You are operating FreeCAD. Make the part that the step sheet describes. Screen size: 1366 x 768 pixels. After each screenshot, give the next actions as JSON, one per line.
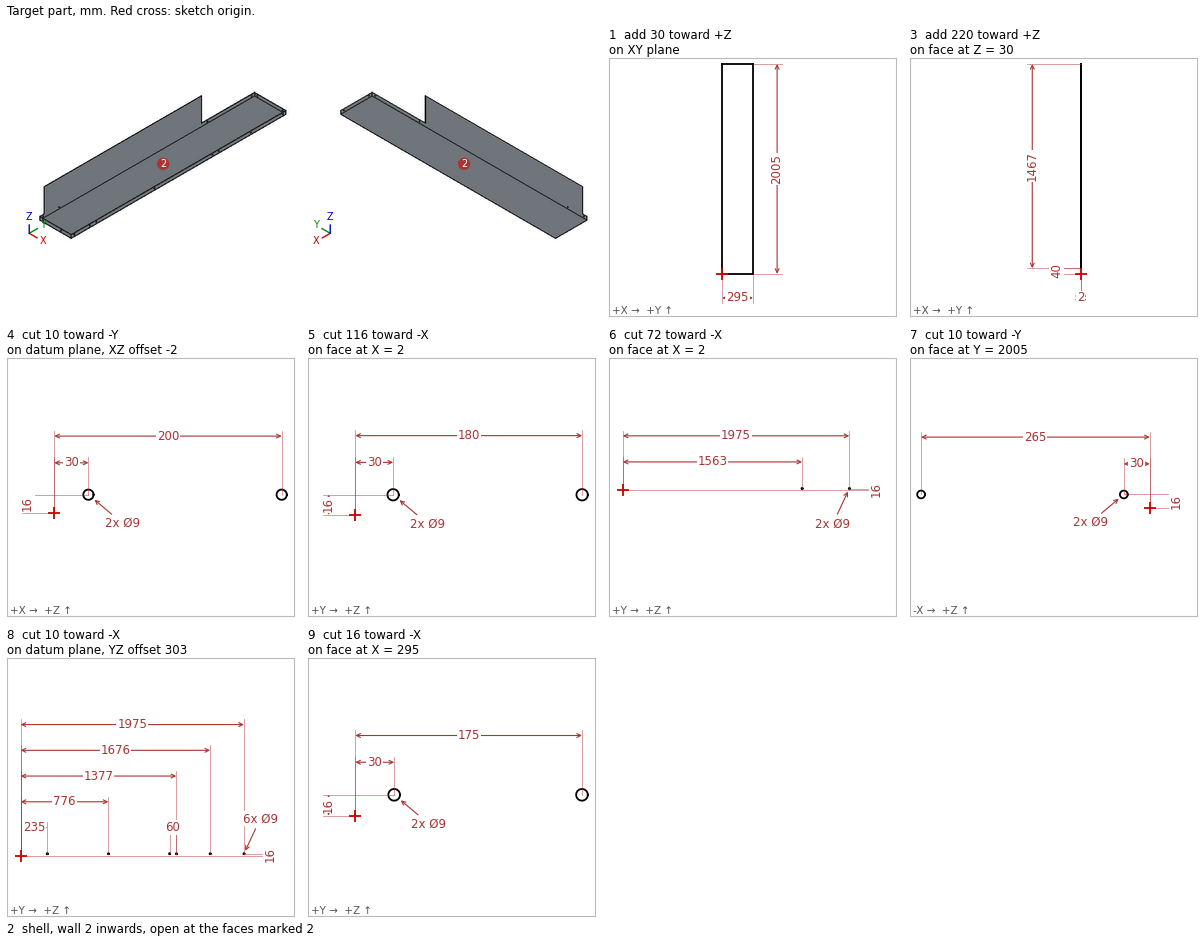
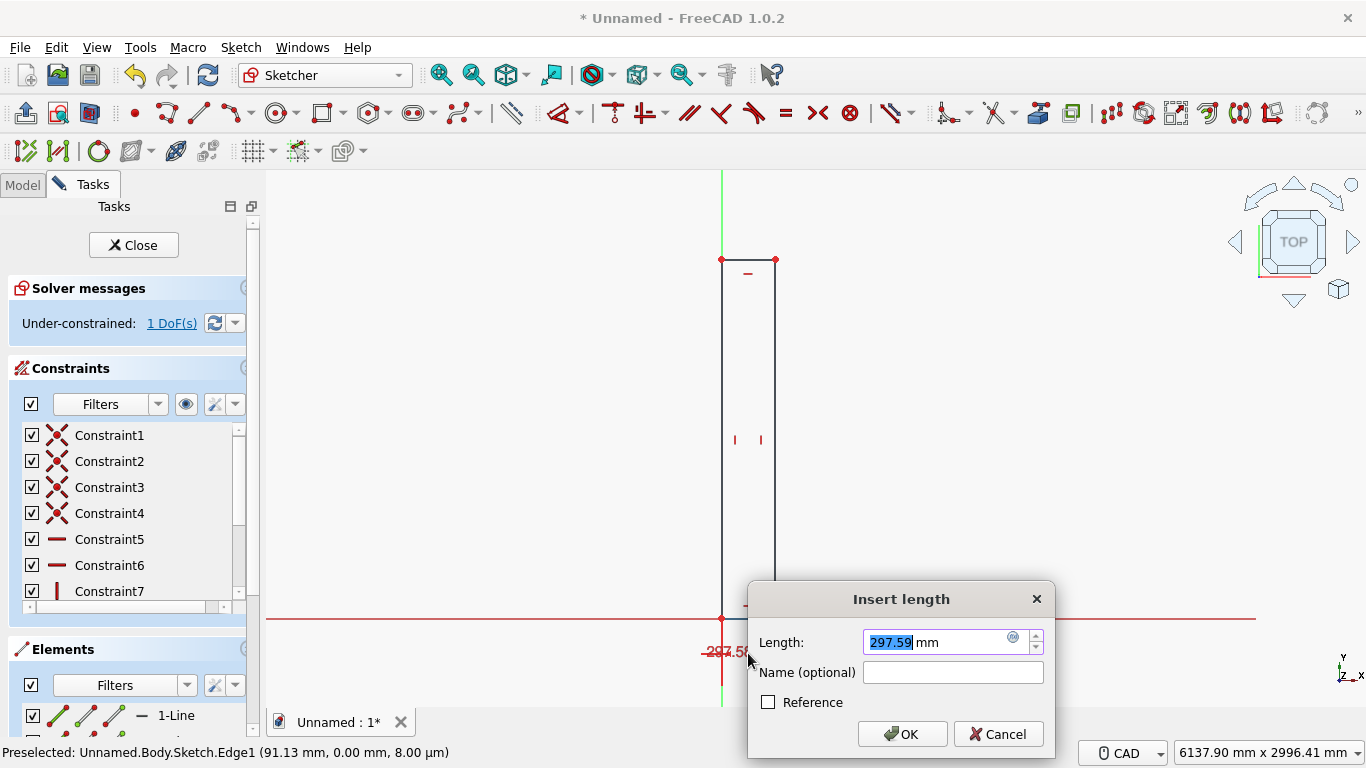
{"action": "type", "text": "295"}
{"action": "key", "text": "Return"}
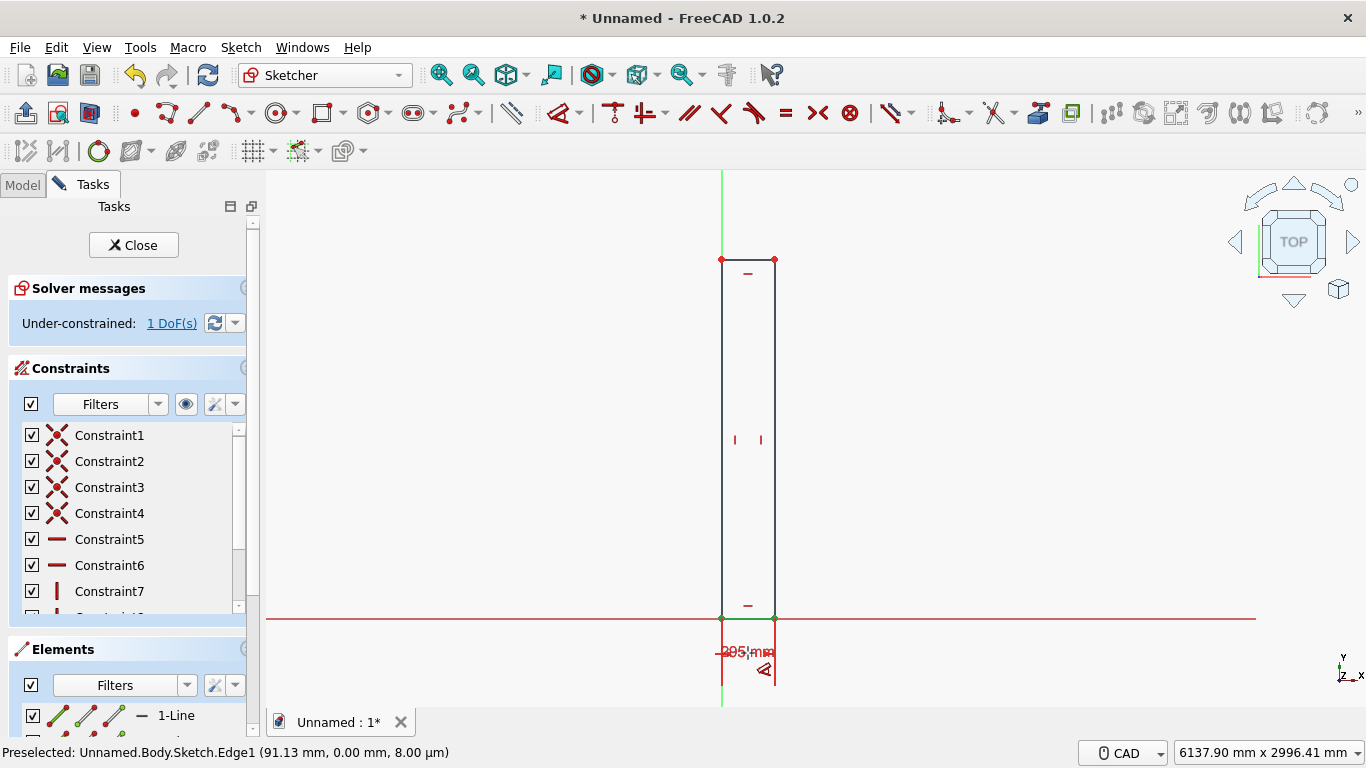
{"action": "left_click", "coordinate": [775, 511]}
{"action": "left_click", "coordinate": [809, 439]}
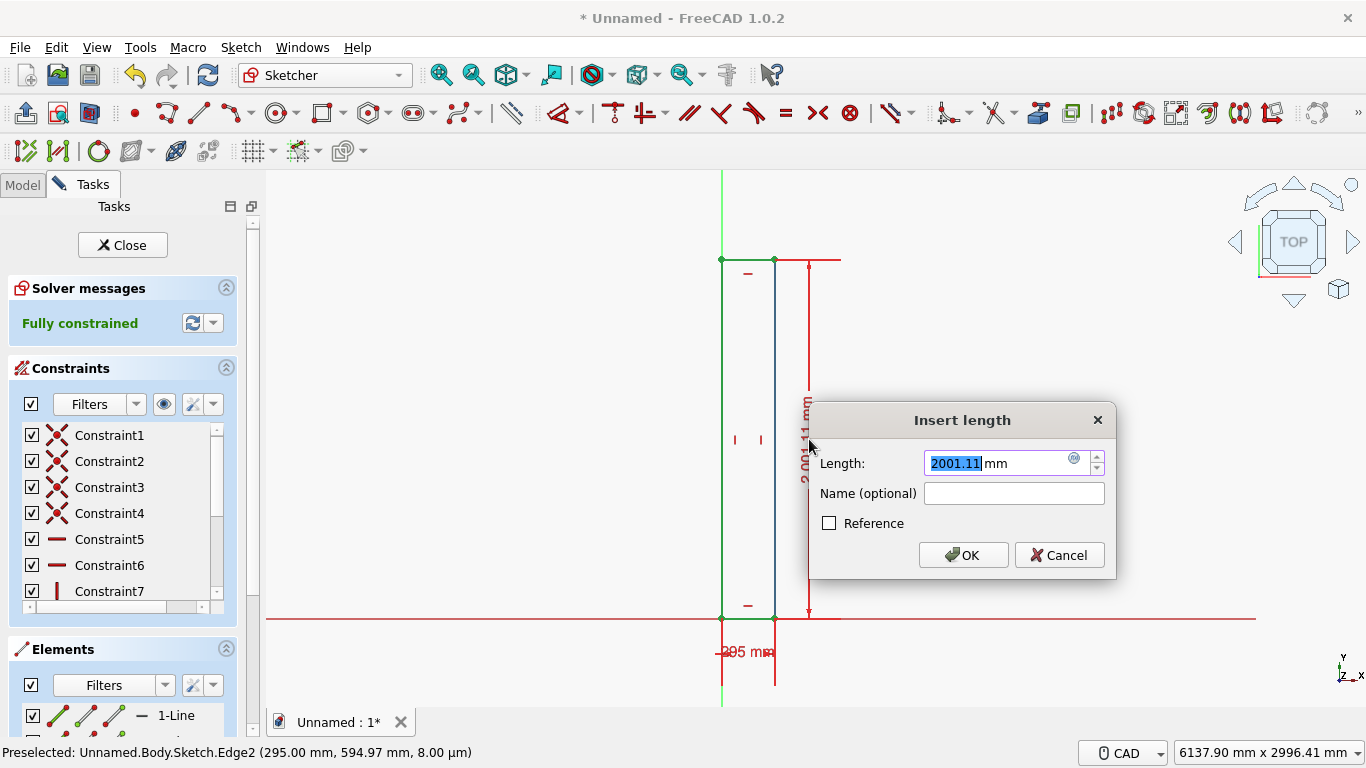
{"action": "type", "text": "2005"}
{"action": "key", "text": "Return"}
{"action": "key", "text": "Escape"}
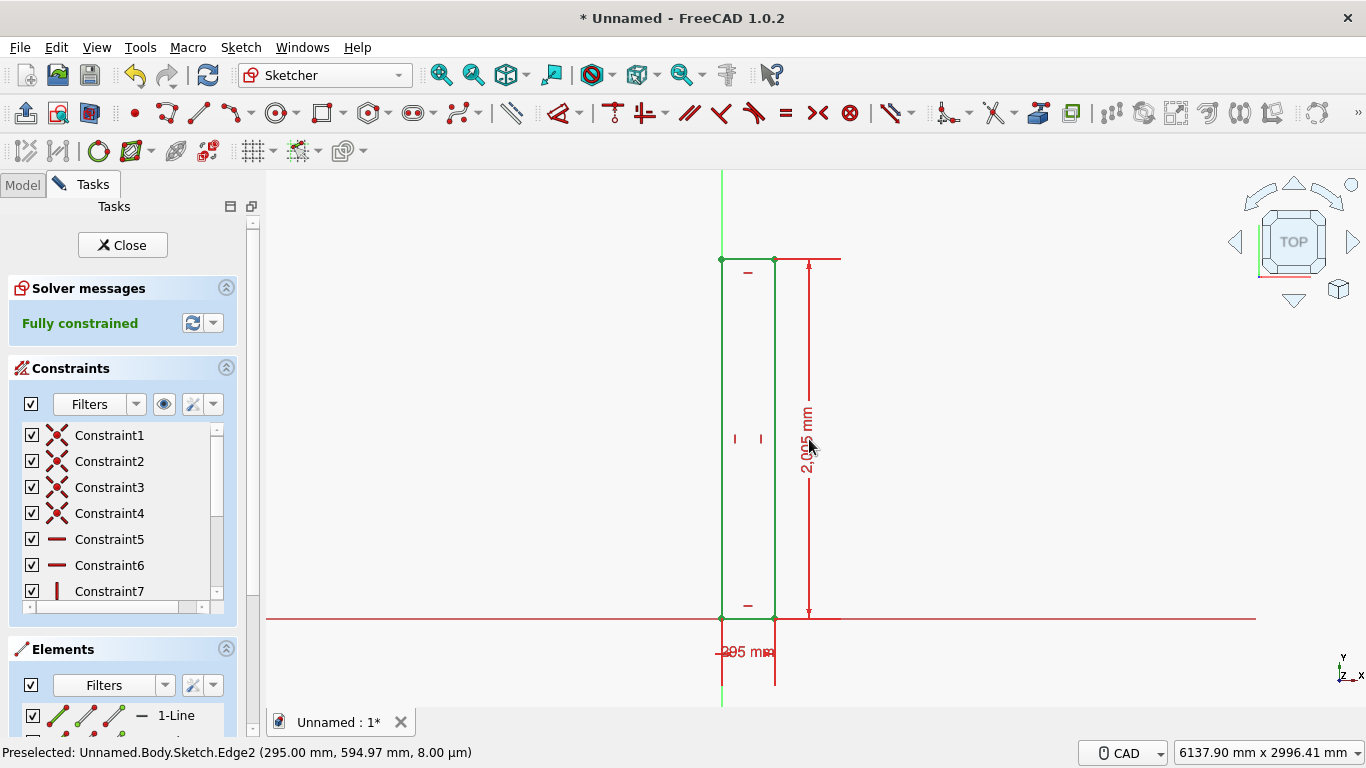
{"action": "left_click", "coordinate": [123, 245]}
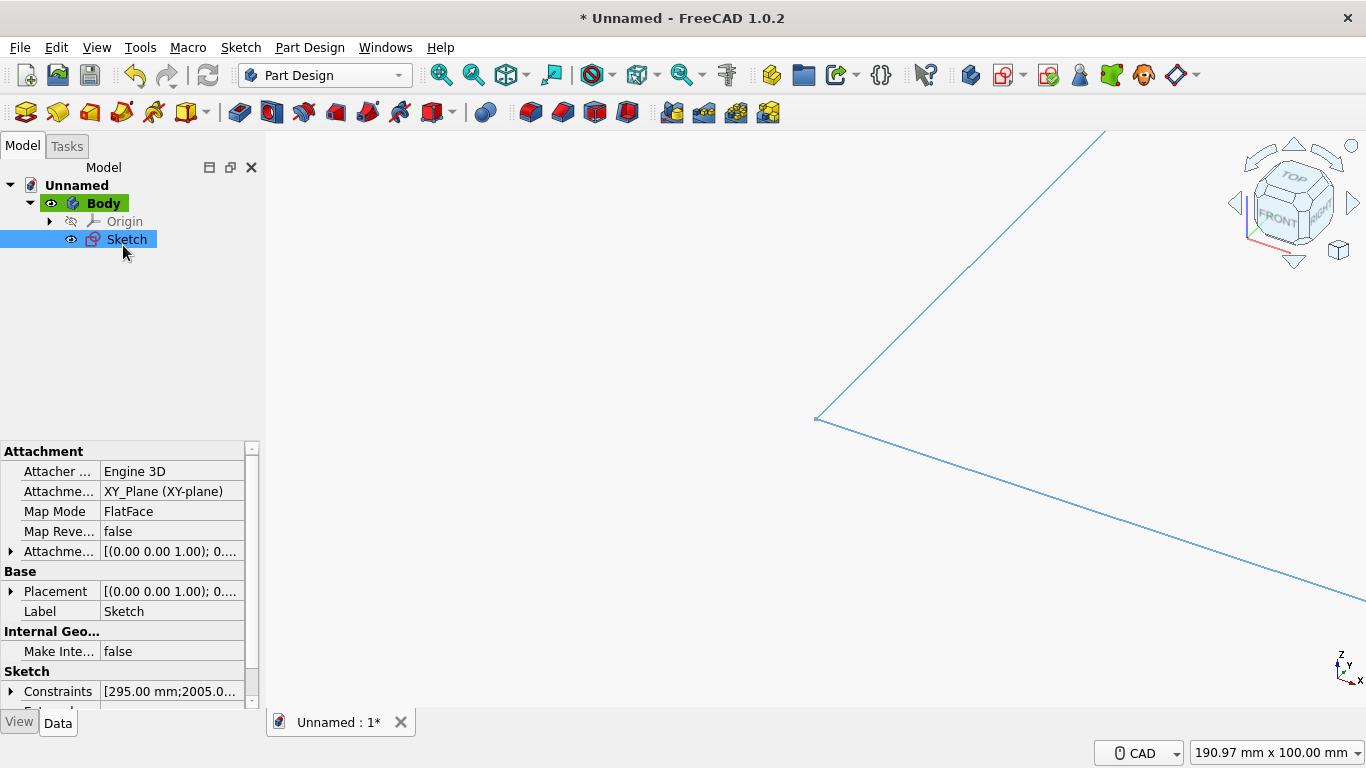
{"action": "left_click", "coordinate": [26, 112]}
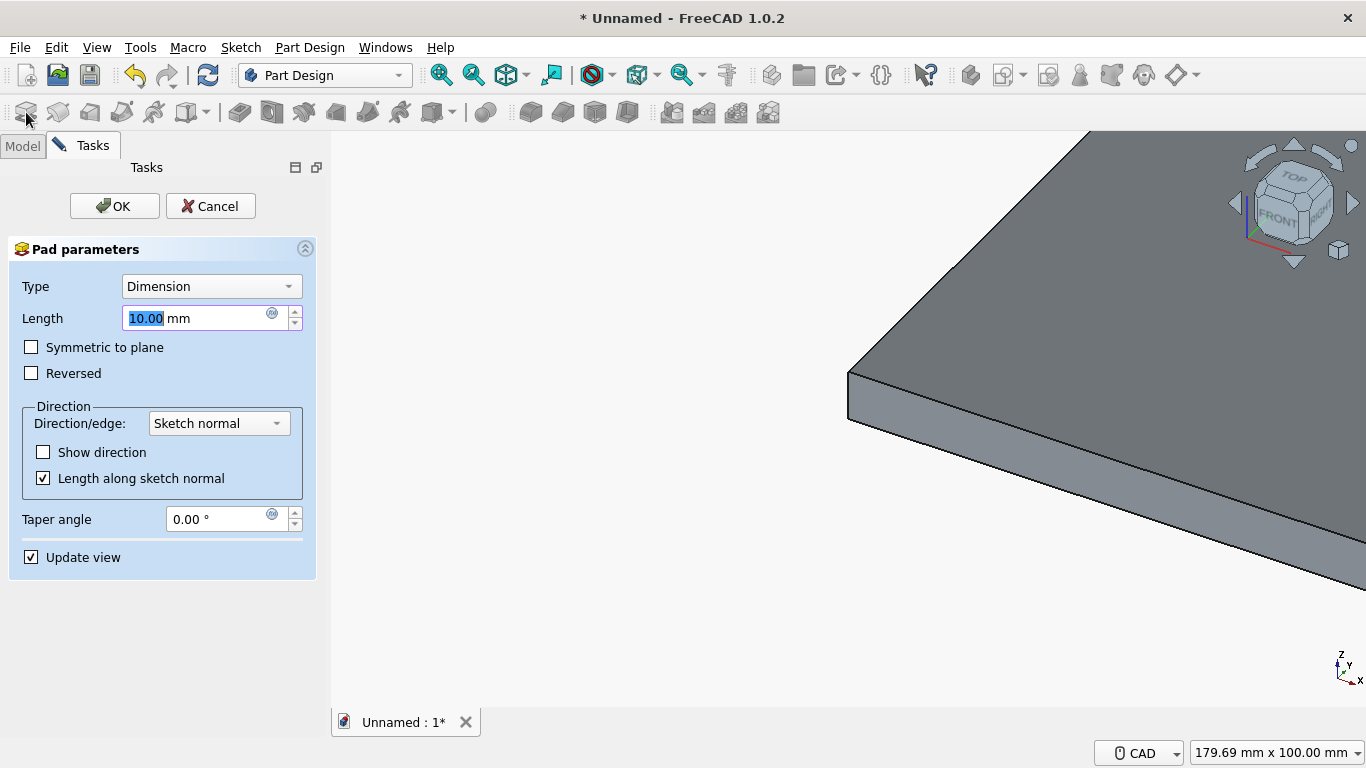
{"action": "type", "text": "30"}
{"action": "key", "text": "Tab"}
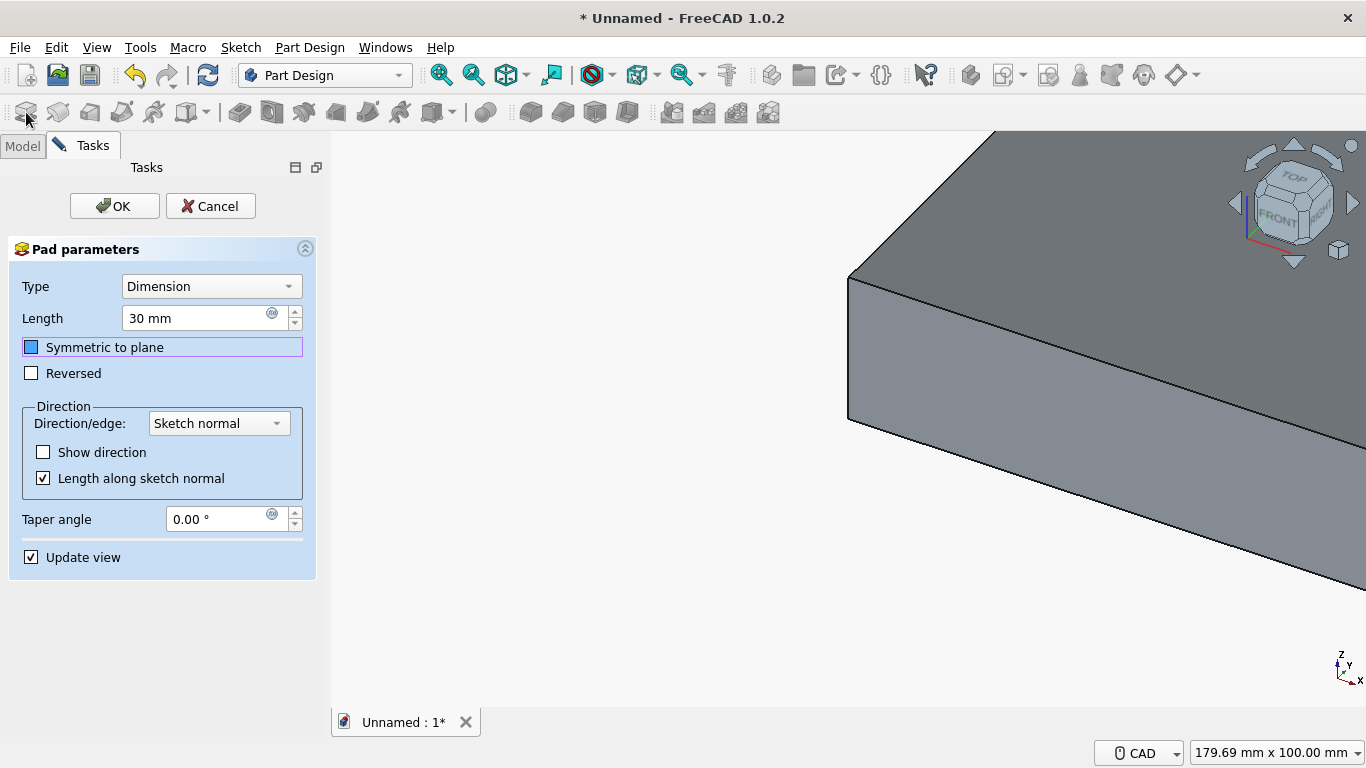
{"action": "left_click", "coordinate": [115, 206]}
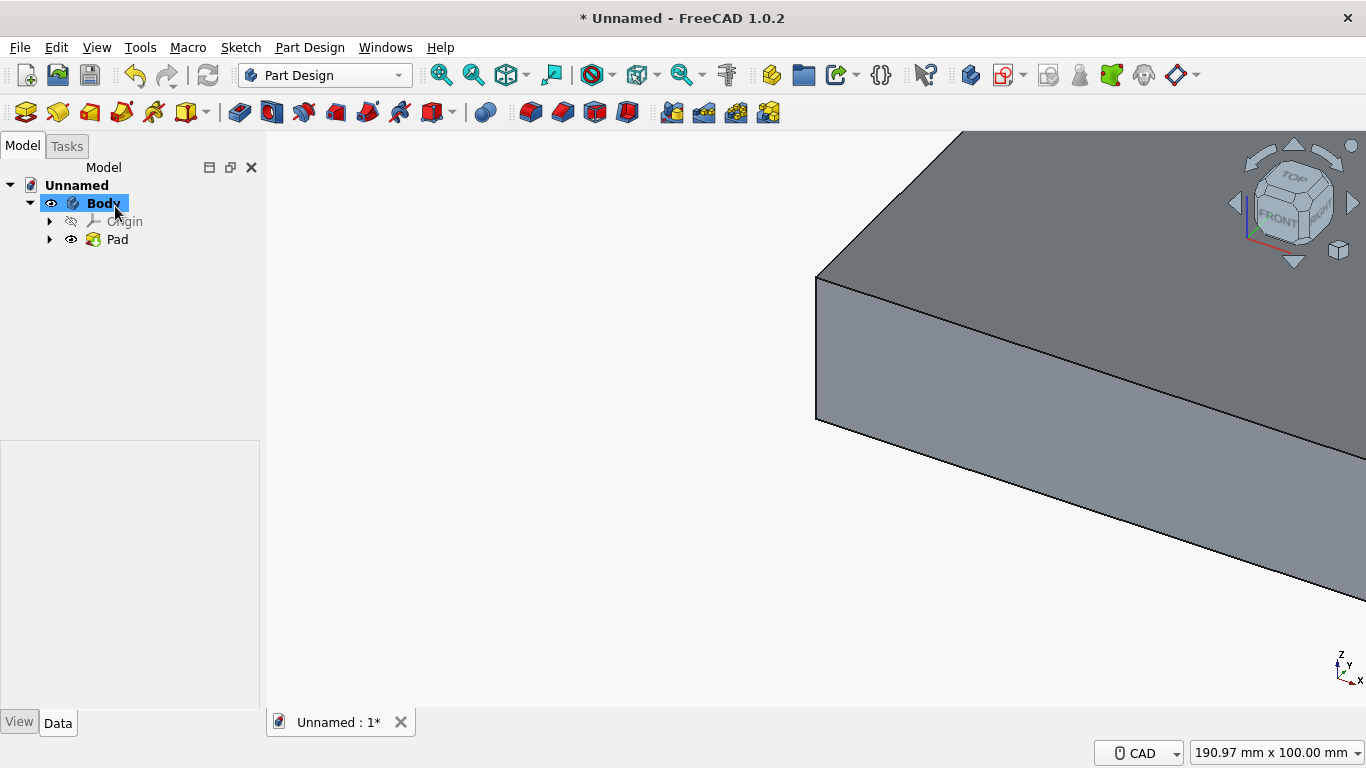
{"action": "left_click", "coordinate": [442, 76]}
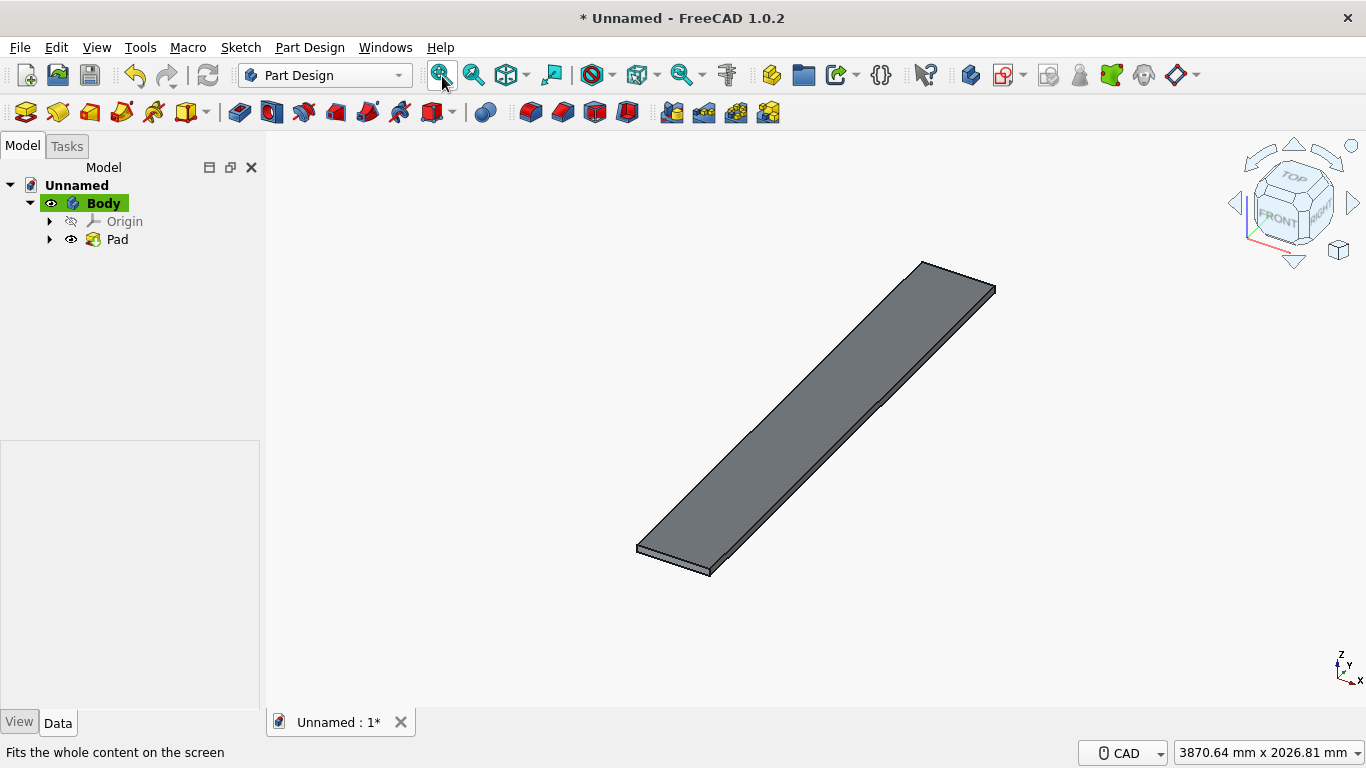
{"action": "left_click", "coordinate": [897, 334]}